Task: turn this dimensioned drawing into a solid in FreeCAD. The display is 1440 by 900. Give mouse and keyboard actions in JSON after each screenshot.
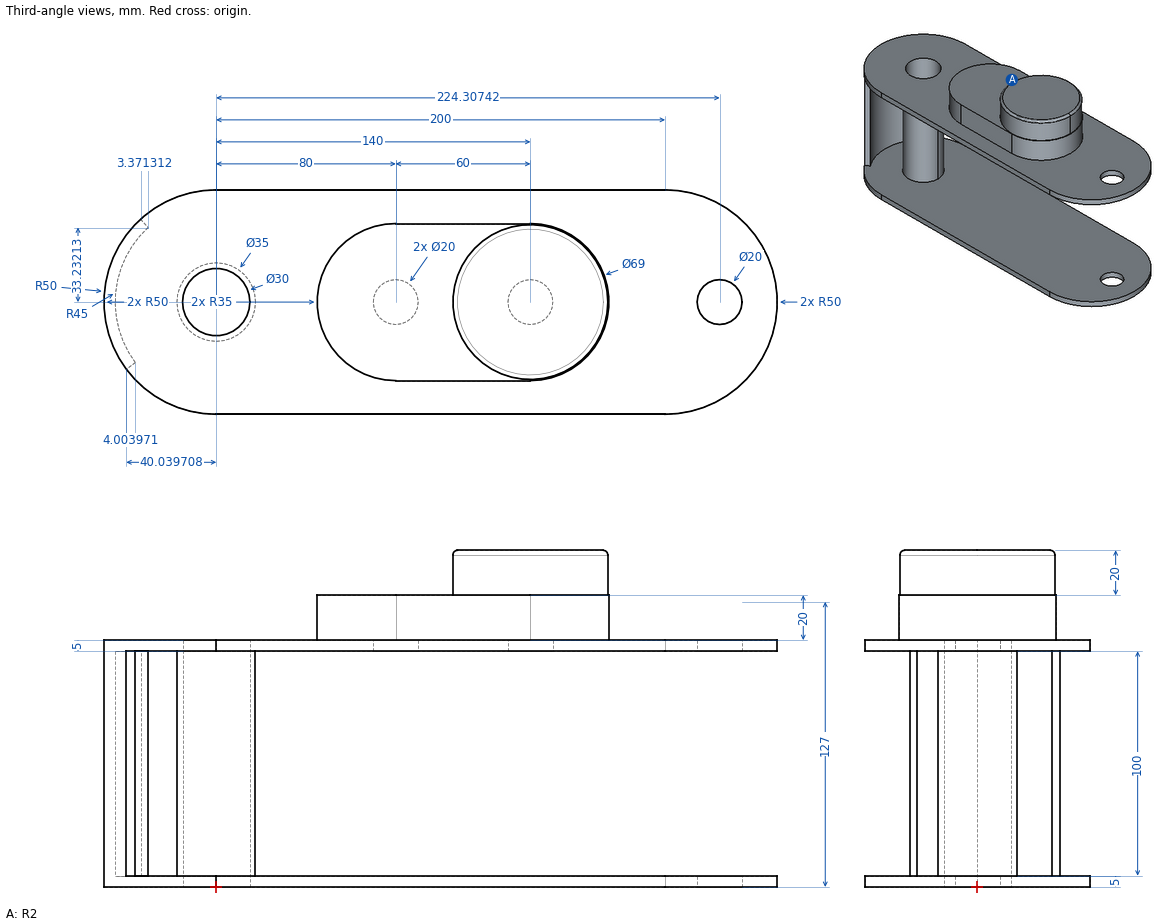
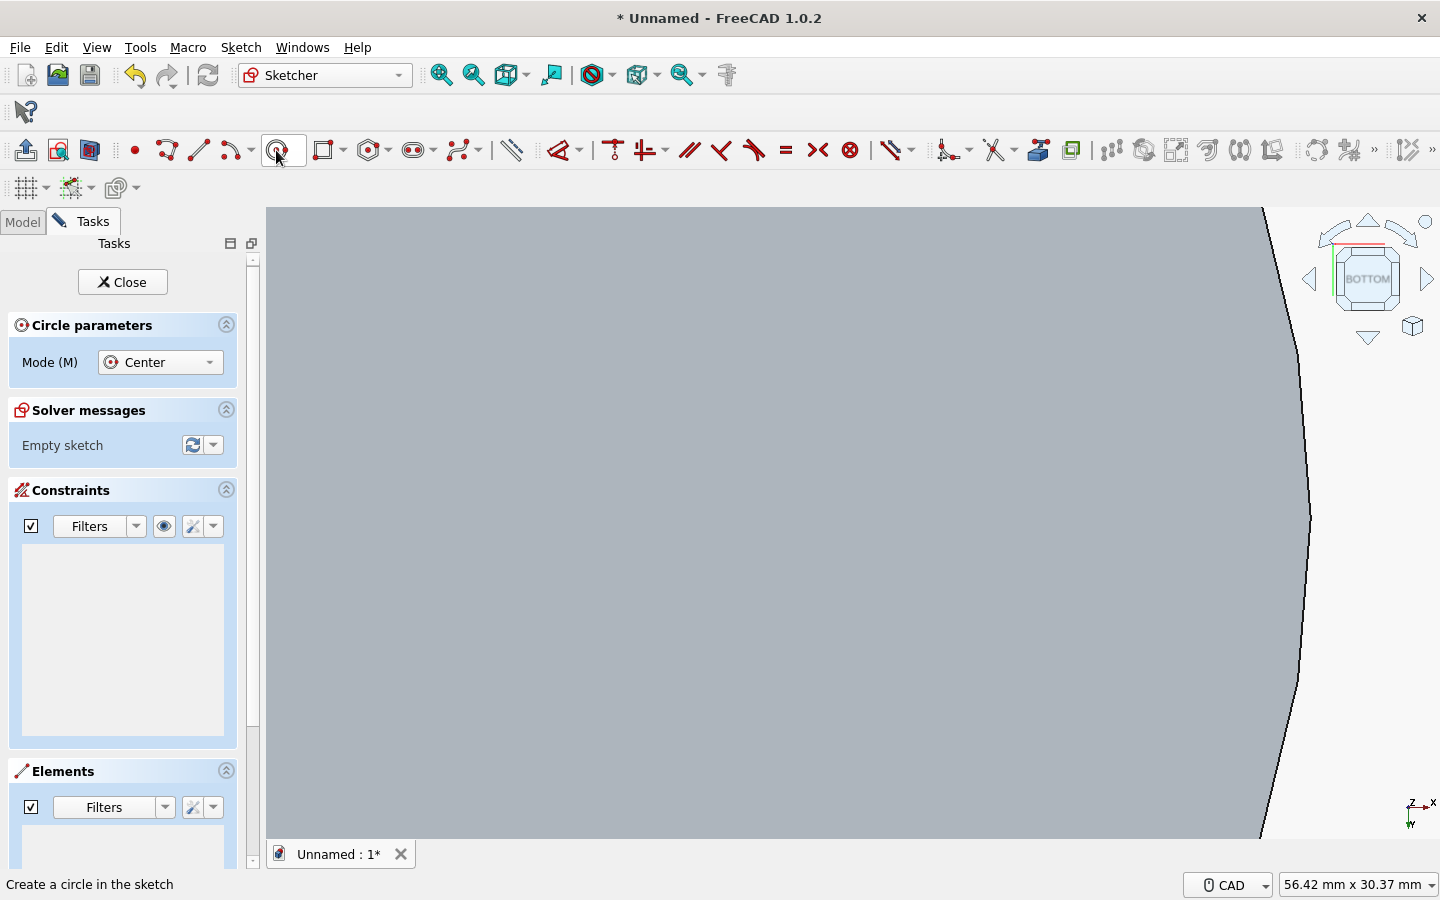
{"action": "left_click", "coordinate": [776, 518]}
{"action": "left_click", "coordinate": [923, 371]}
{"action": "key", "text": "Escape"}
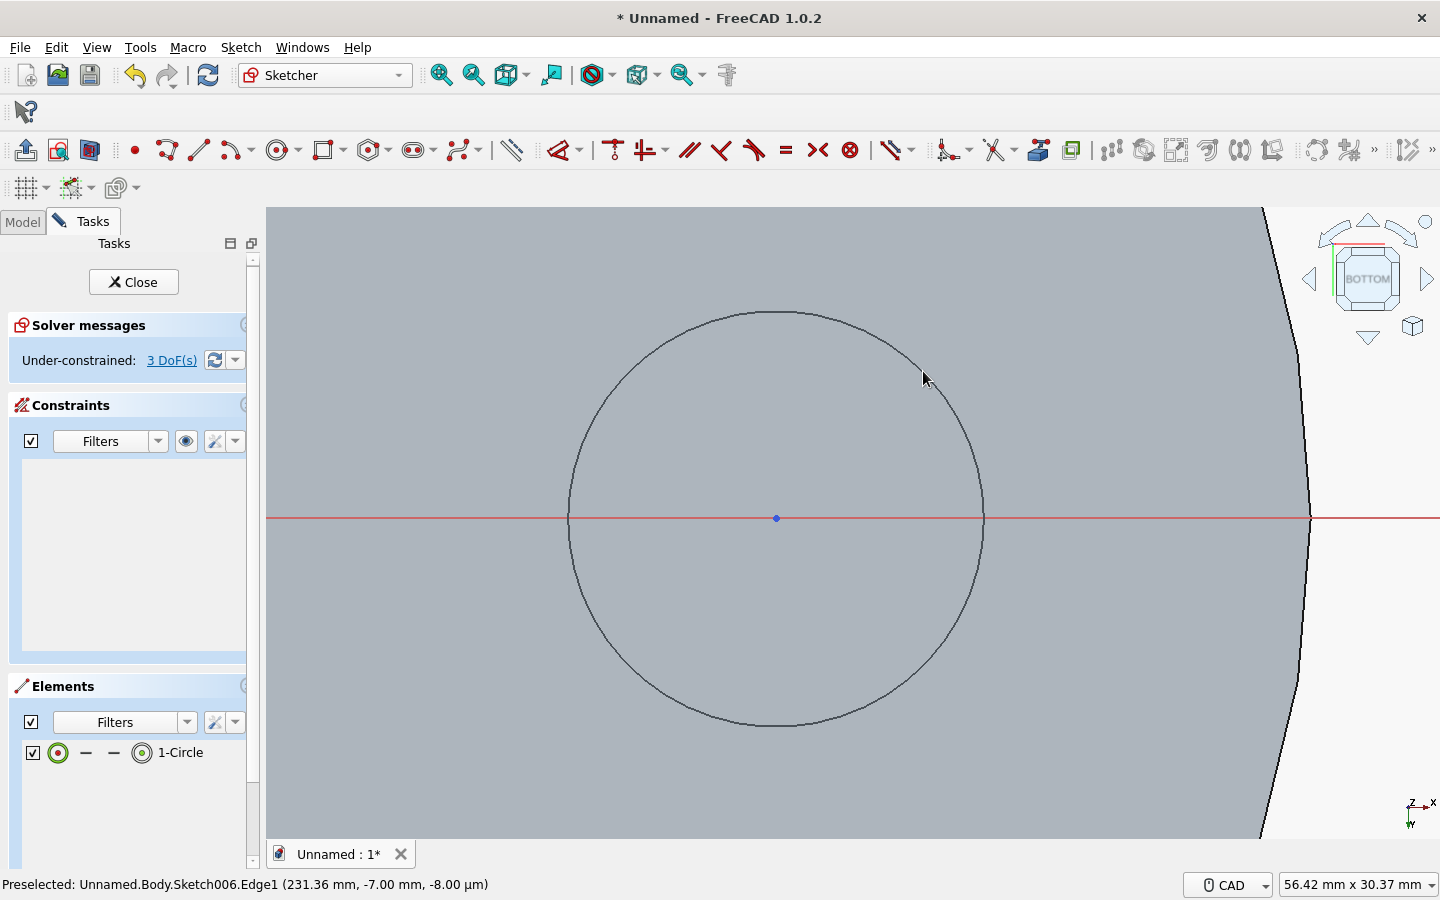
{"action": "left_click", "coordinate": [776, 519]}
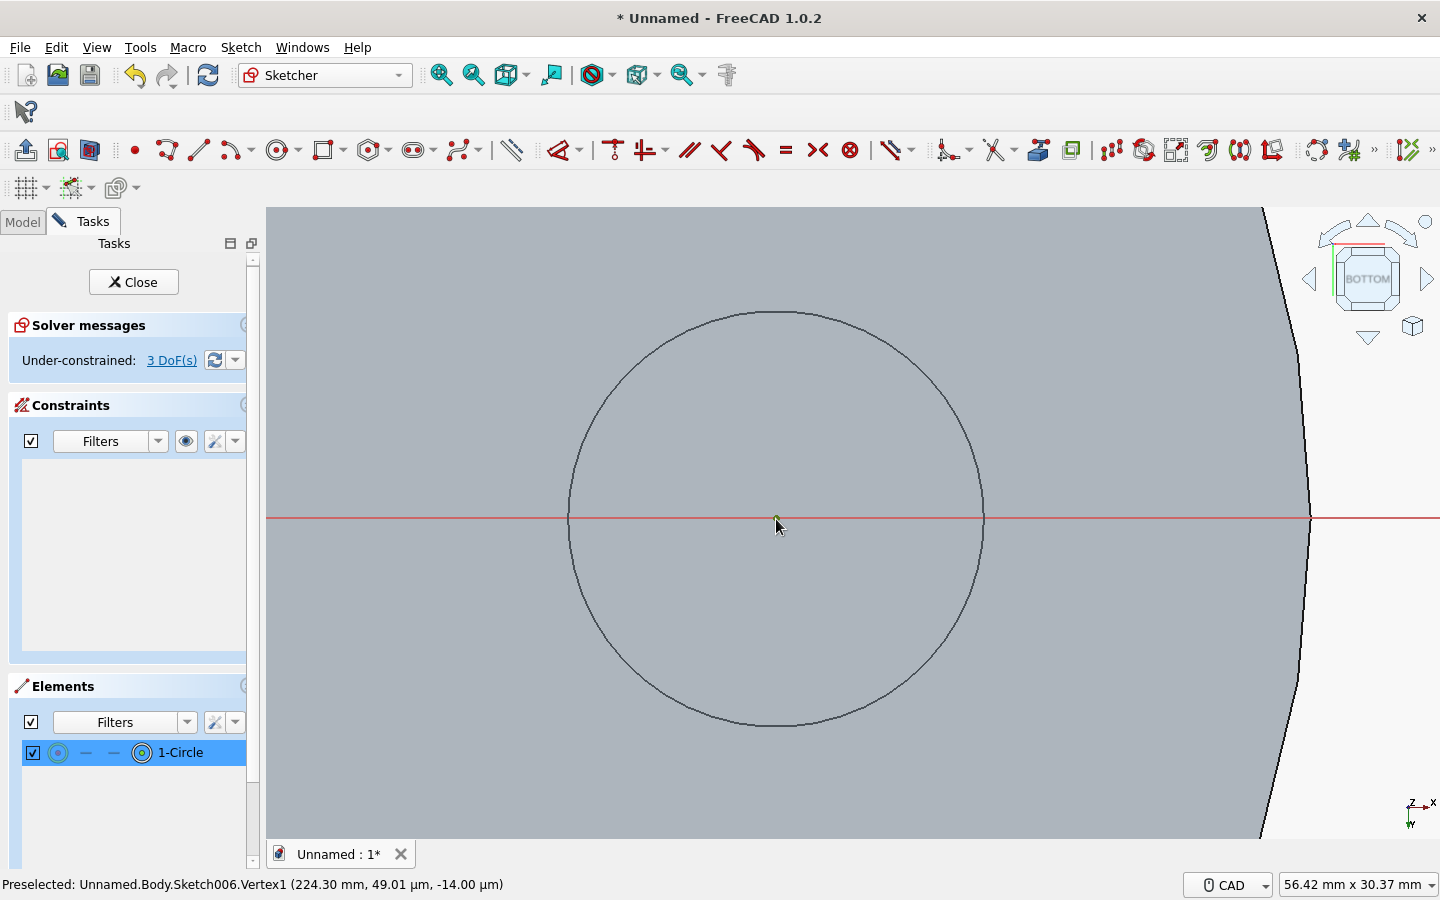
{"action": "left_click", "coordinate": [364, 518]}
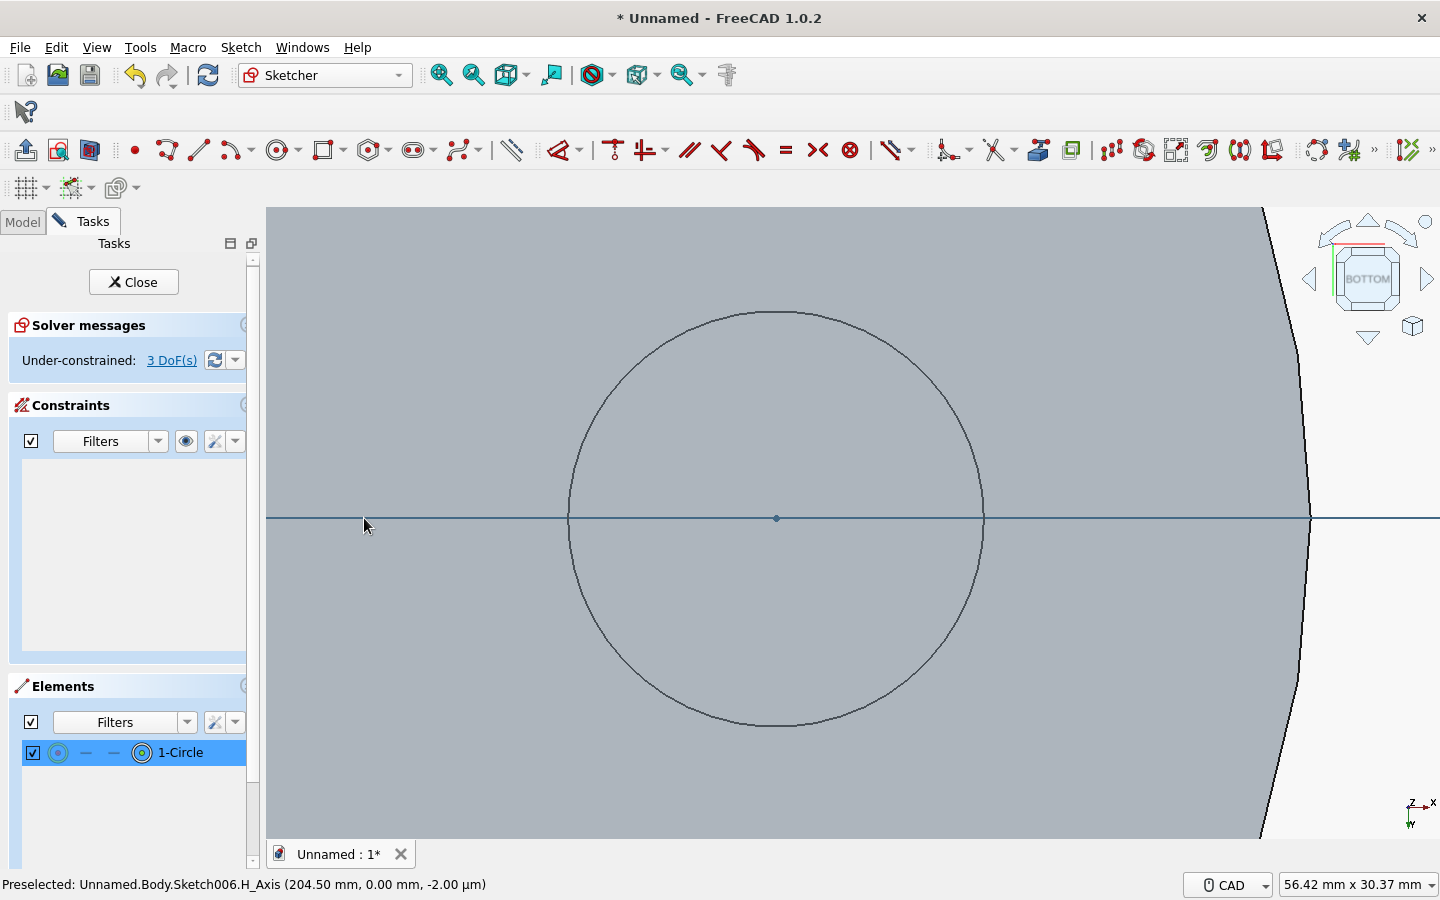
{"action": "left_click", "coordinate": [614, 150]}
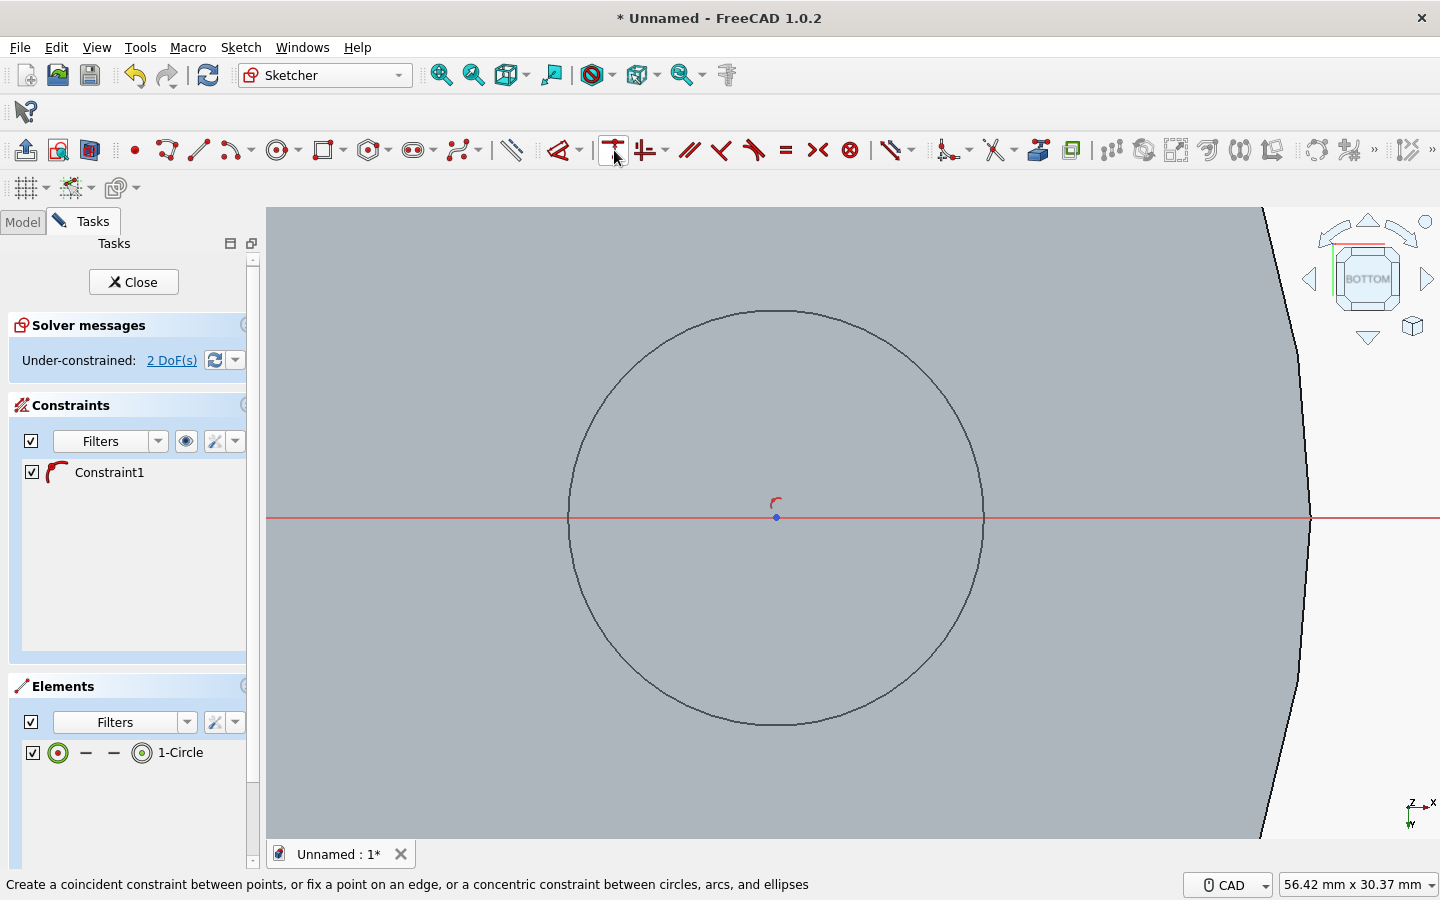
{"action": "left_click", "coordinate": [558, 150]}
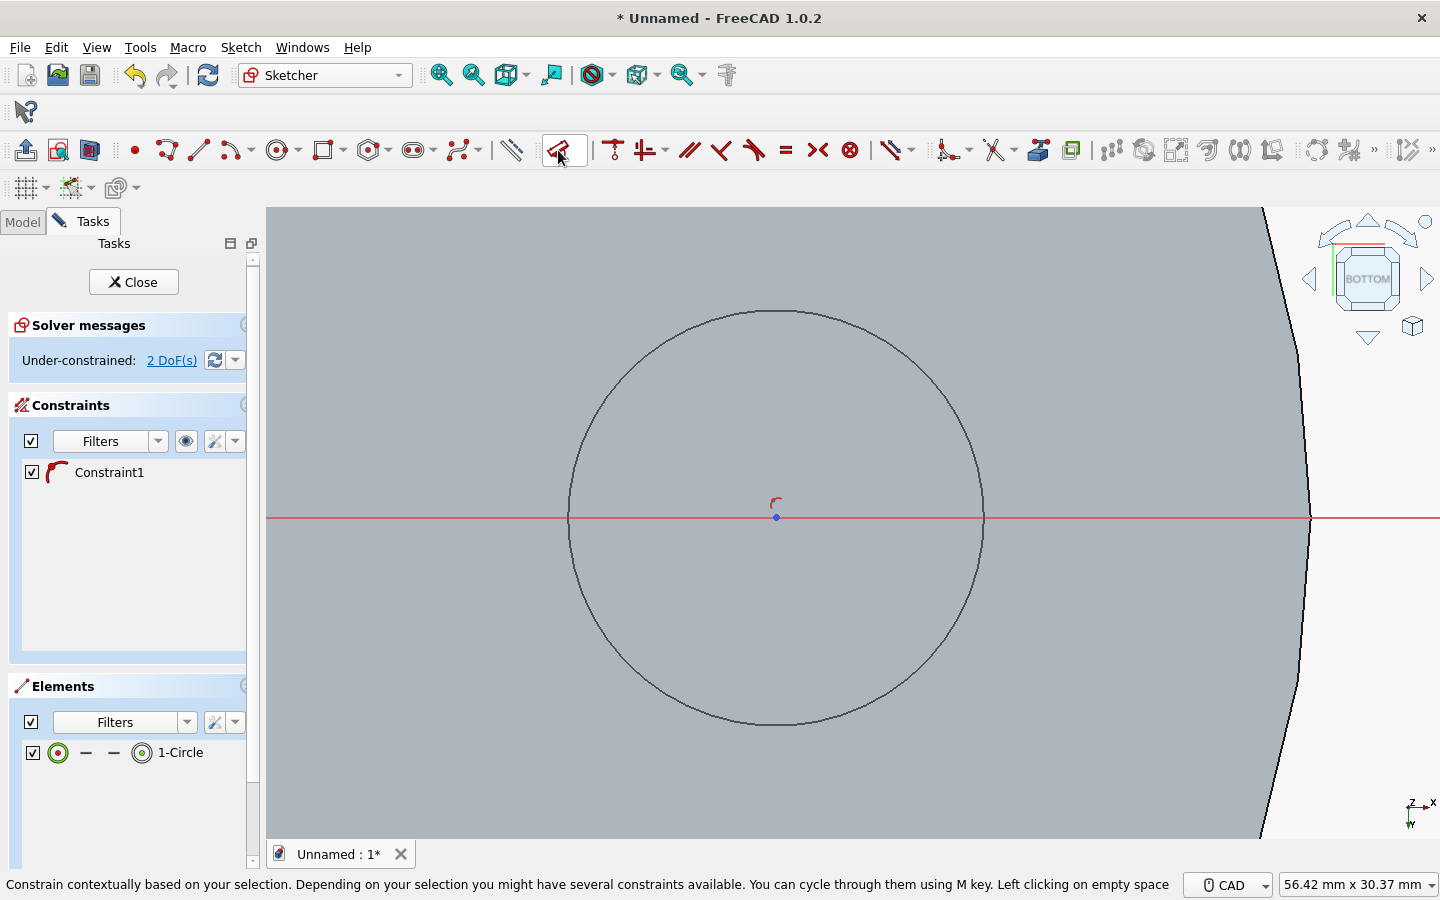
{"action": "left_click", "coordinate": [923, 371]}
{"action": "left_click", "coordinate": [946, 348]}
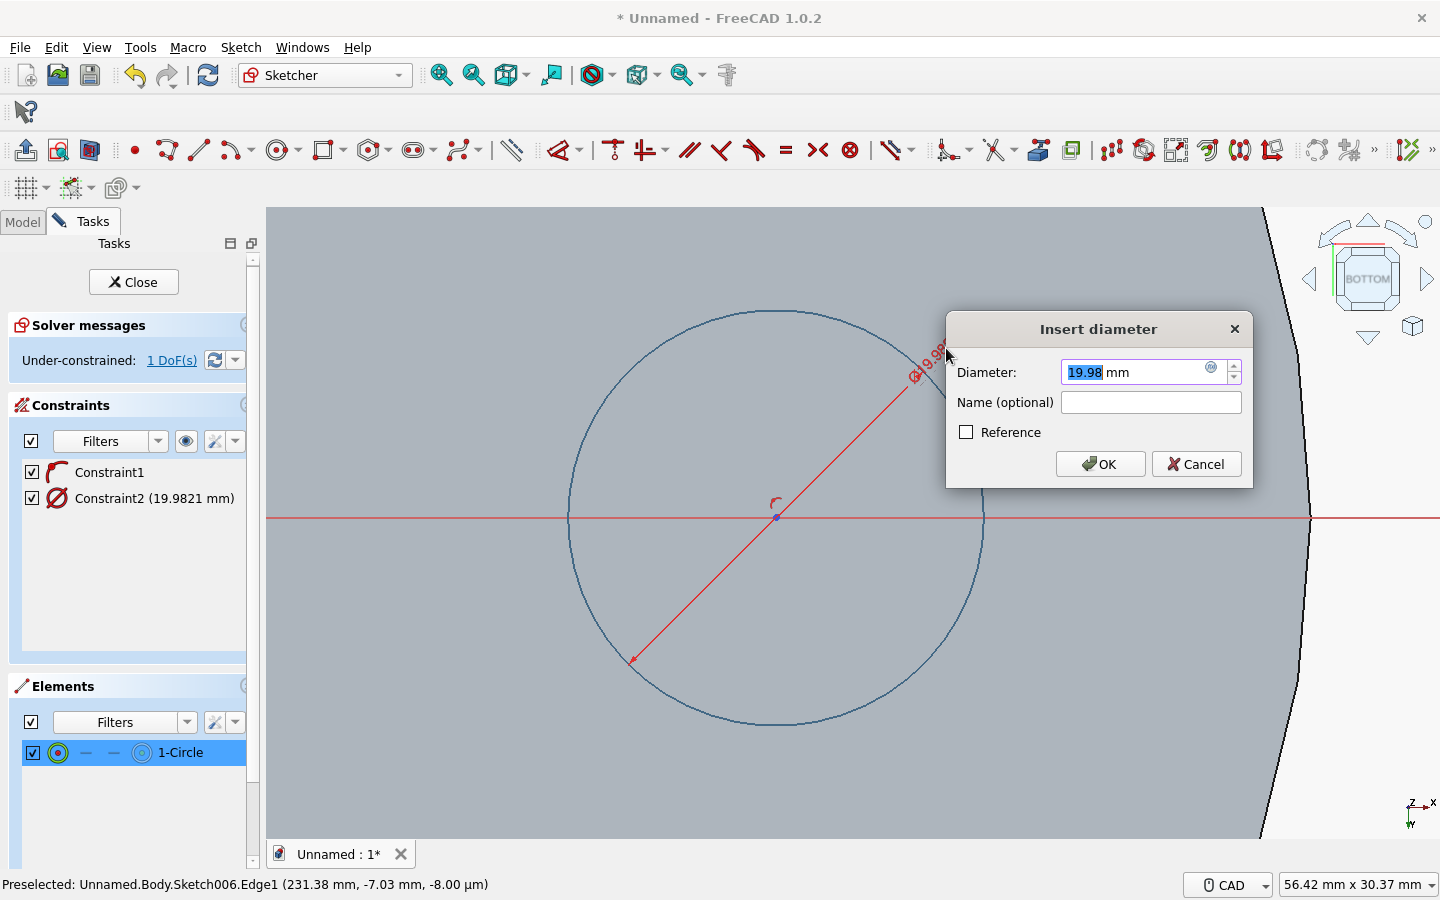
{"action": "type", "text": "20"}
{"action": "key", "text": "Return"}